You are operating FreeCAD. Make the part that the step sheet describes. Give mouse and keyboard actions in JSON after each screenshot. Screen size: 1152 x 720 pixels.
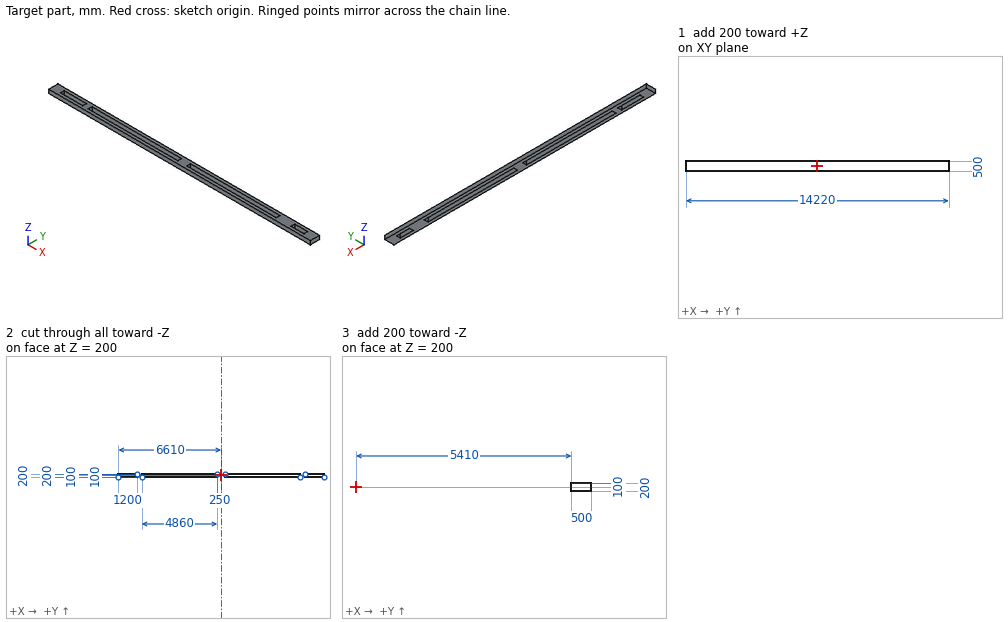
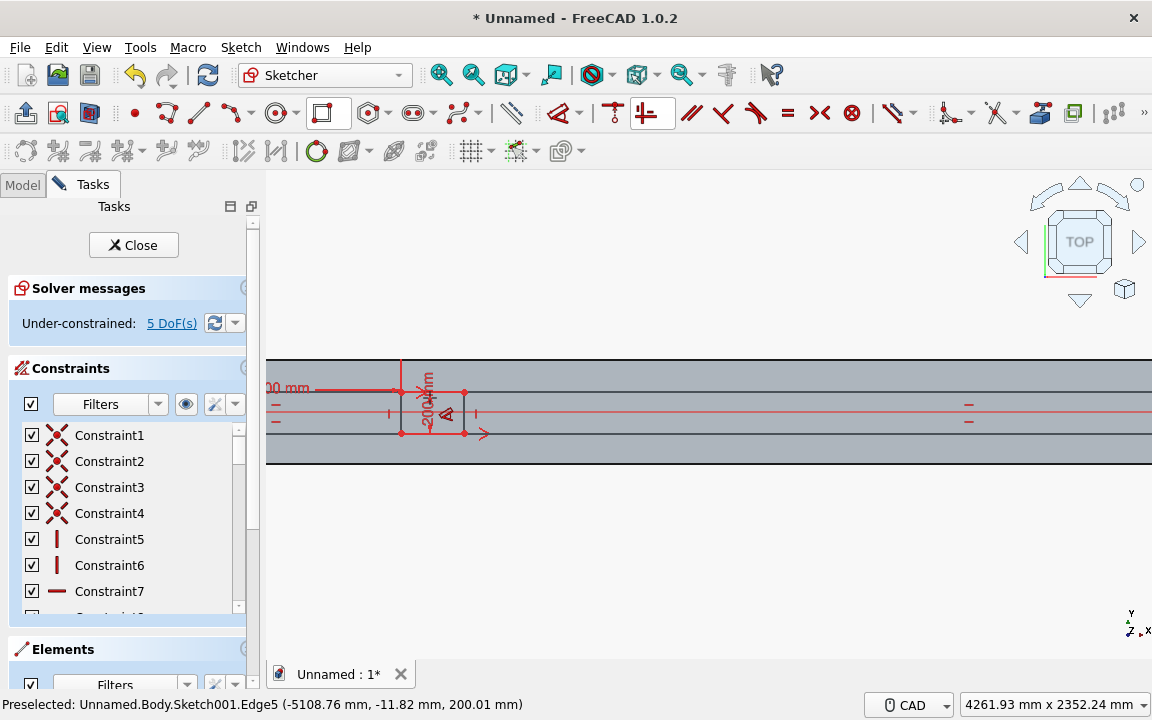
{"action": "left_click", "coordinate": [767, 434]}
{"action": "left_click", "coordinate": [726, 468]}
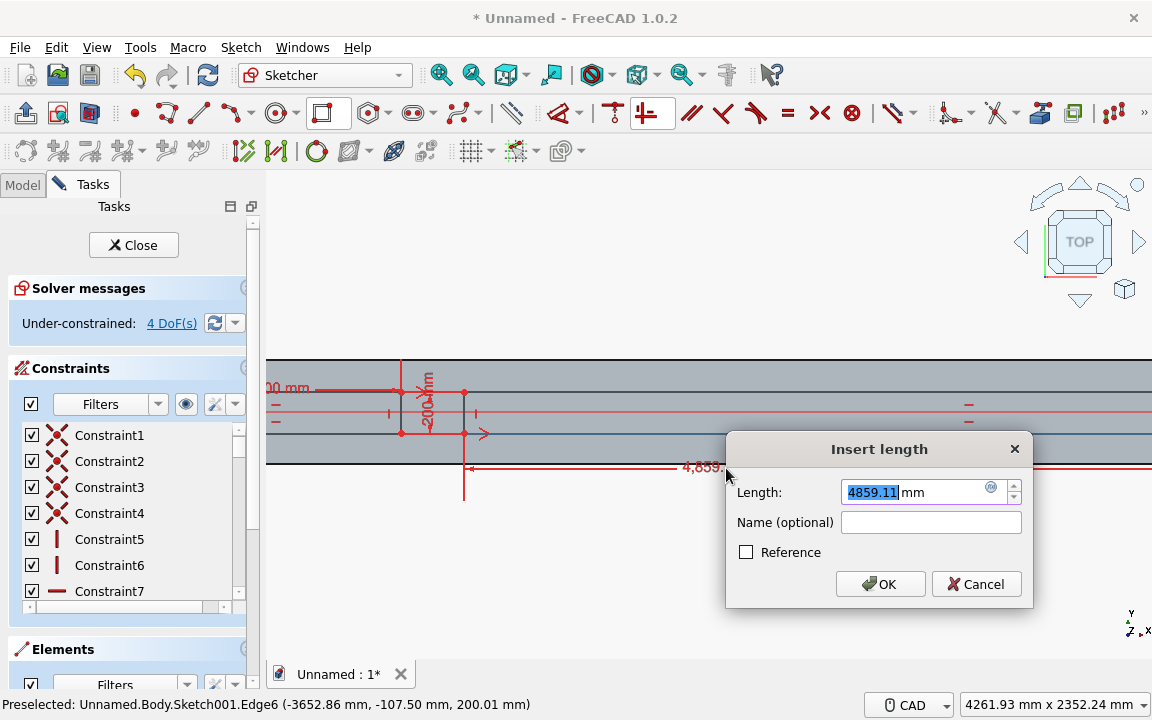
{"action": "type", "text": "4860"}
{"action": "key", "text": "Return"}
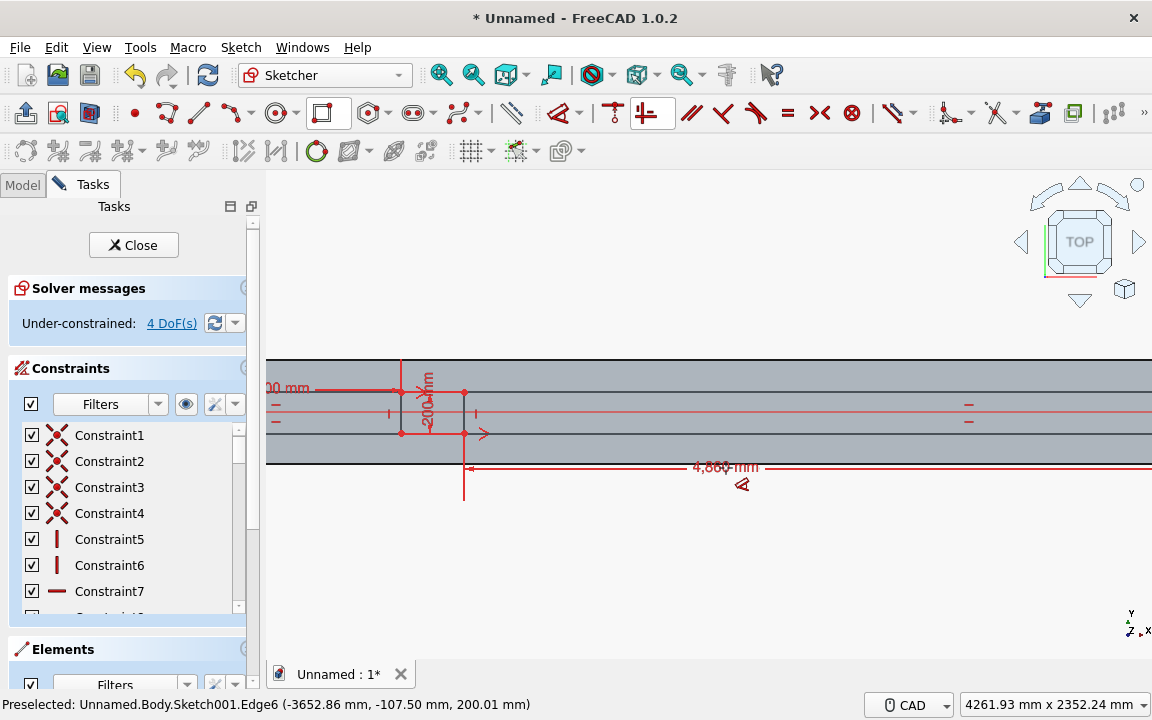
{"action": "scroll", "coordinate": [465, 415], "scroll_direction": "down", "scroll_amount": 9}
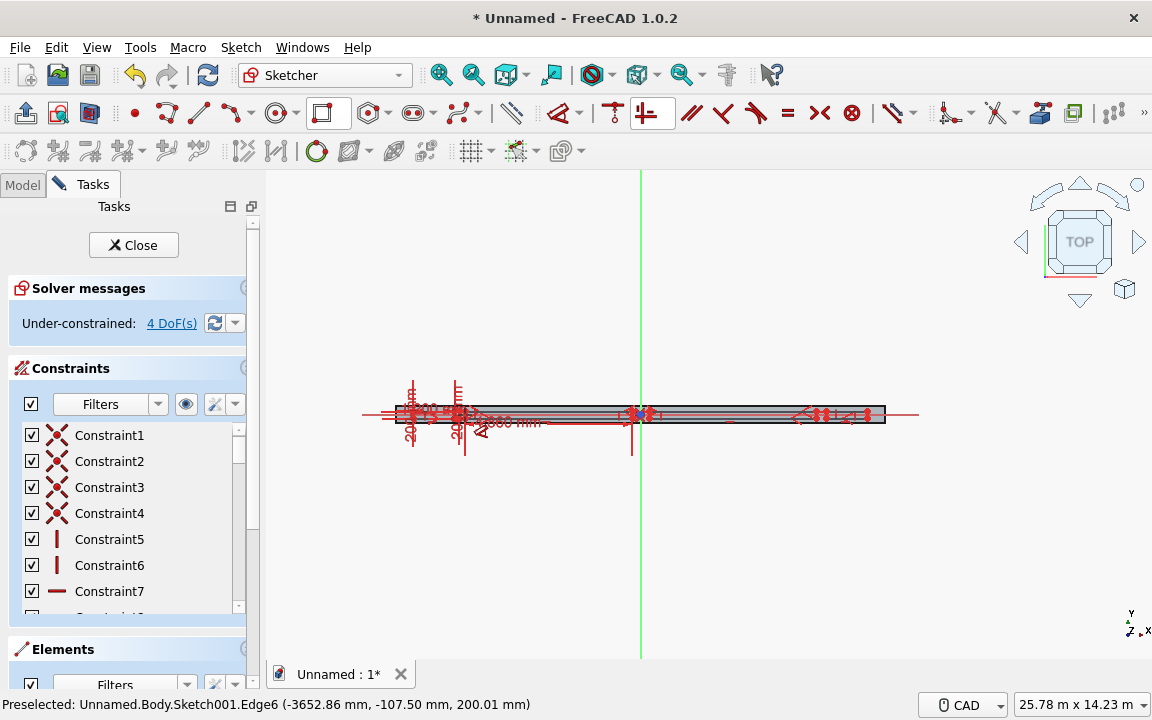
{"action": "scroll", "coordinate": [413, 412], "scroll_direction": "up", "scroll_amount": 13}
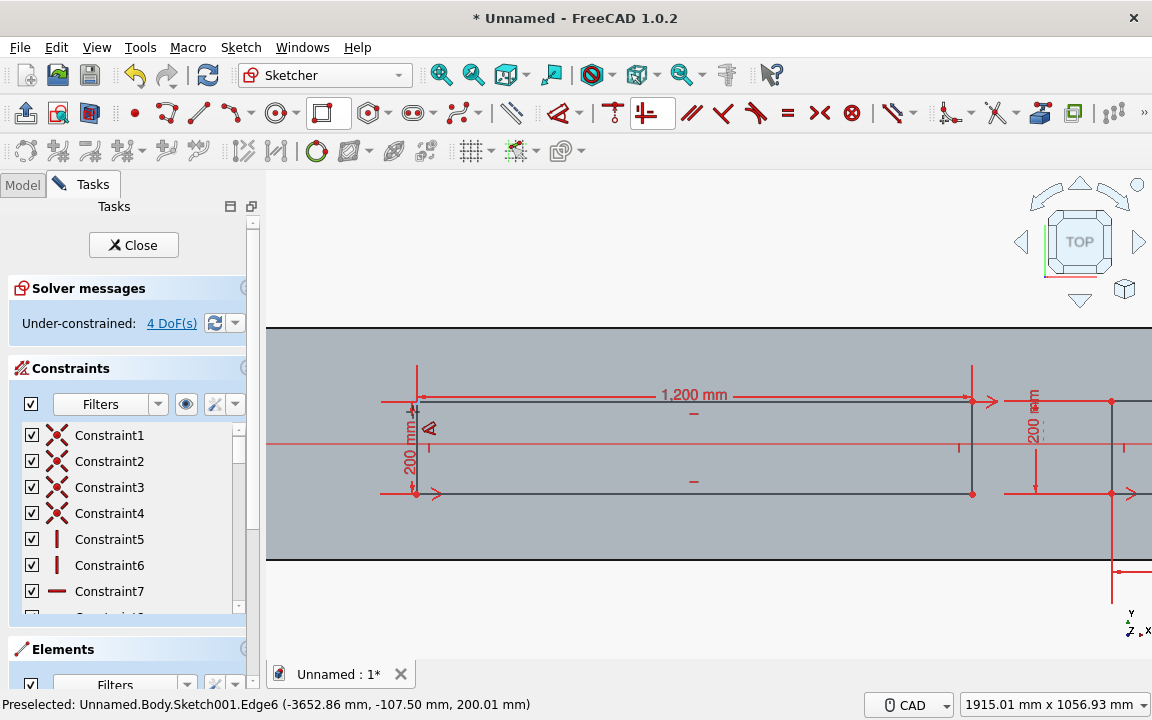
{"action": "left_click", "coordinate": [417, 402]}
{"action": "left_click", "coordinate": [383, 423]}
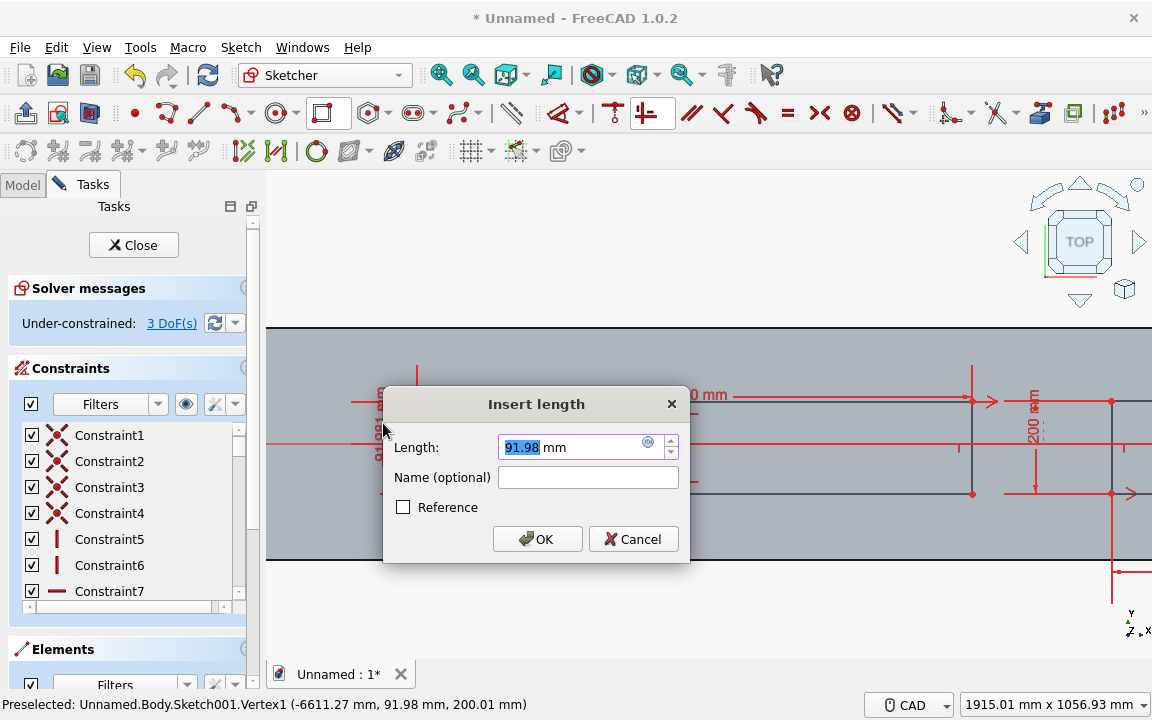
{"action": "type", "text": "100"}
{"action": "key", "text": "Return"}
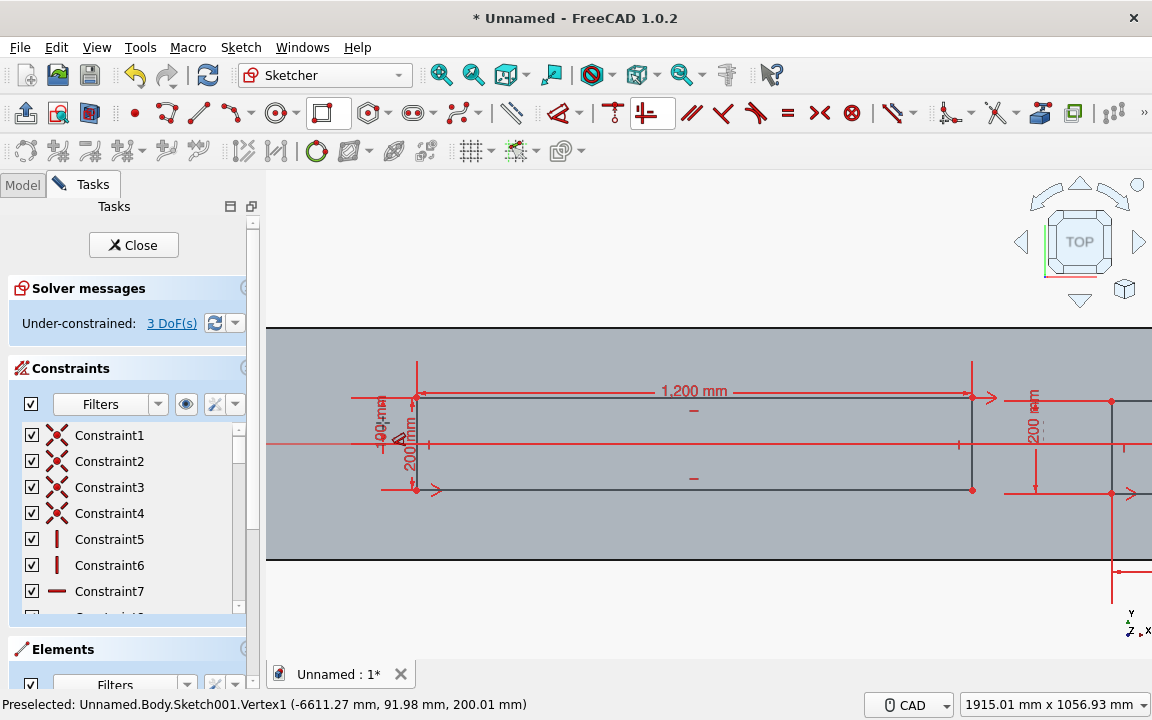
{"action": "scroll", "coordinate": [413, 412], "scroll_direction": "down", "scroll_amount": 13}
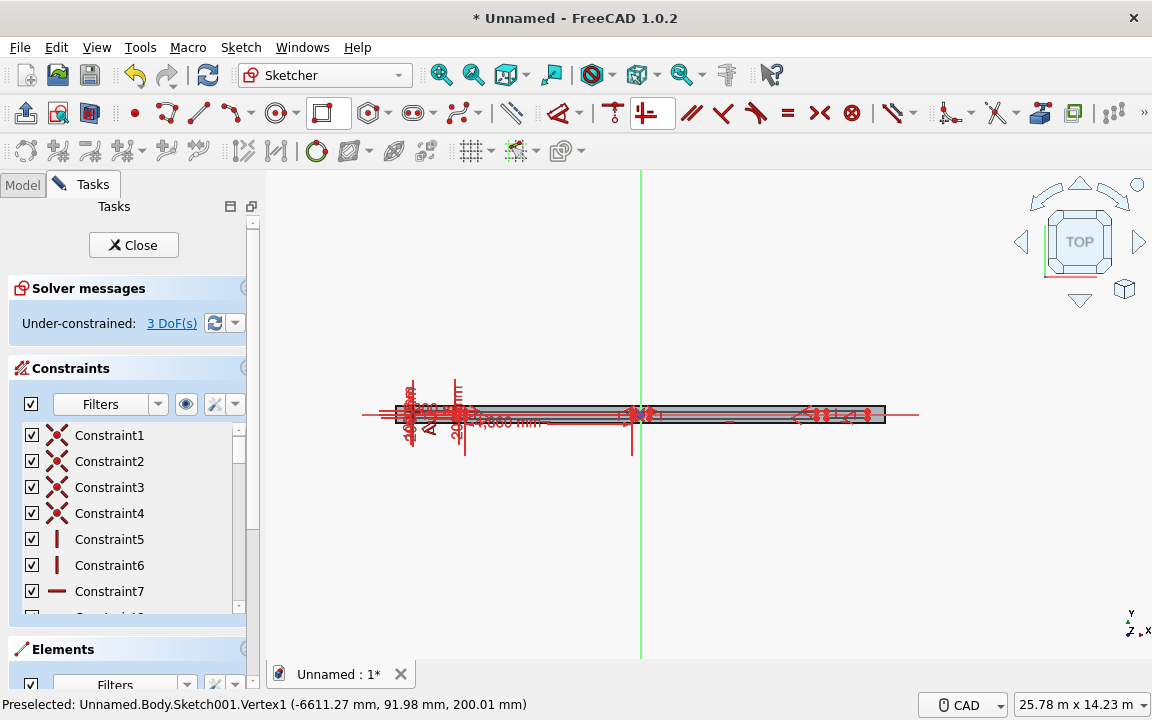
{"action": "scroll", "coordinate": [465, 412], "scroll_direction": "up", "scroll_amount": 13}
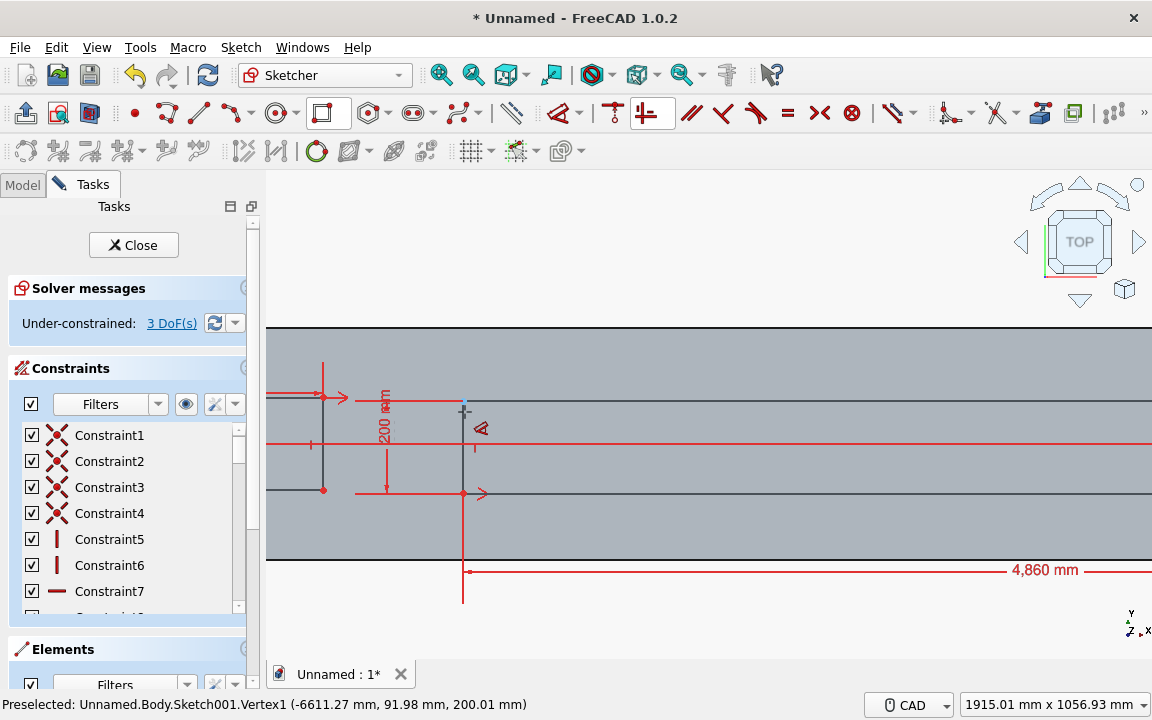
{"action": "left_click", "coordinate": [463, 401]}
{"action": "left_click", "coordinate": [309, 423]}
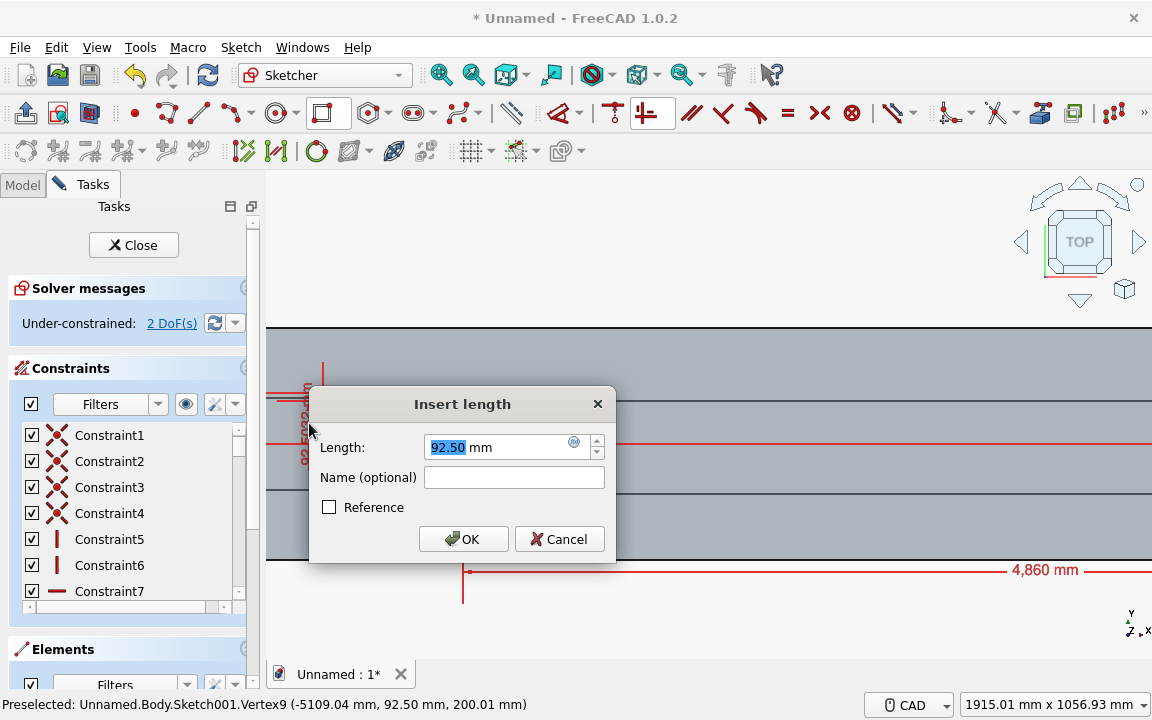
{"action": "type", "text": "100"}
{"action": "key", "text": "Return"}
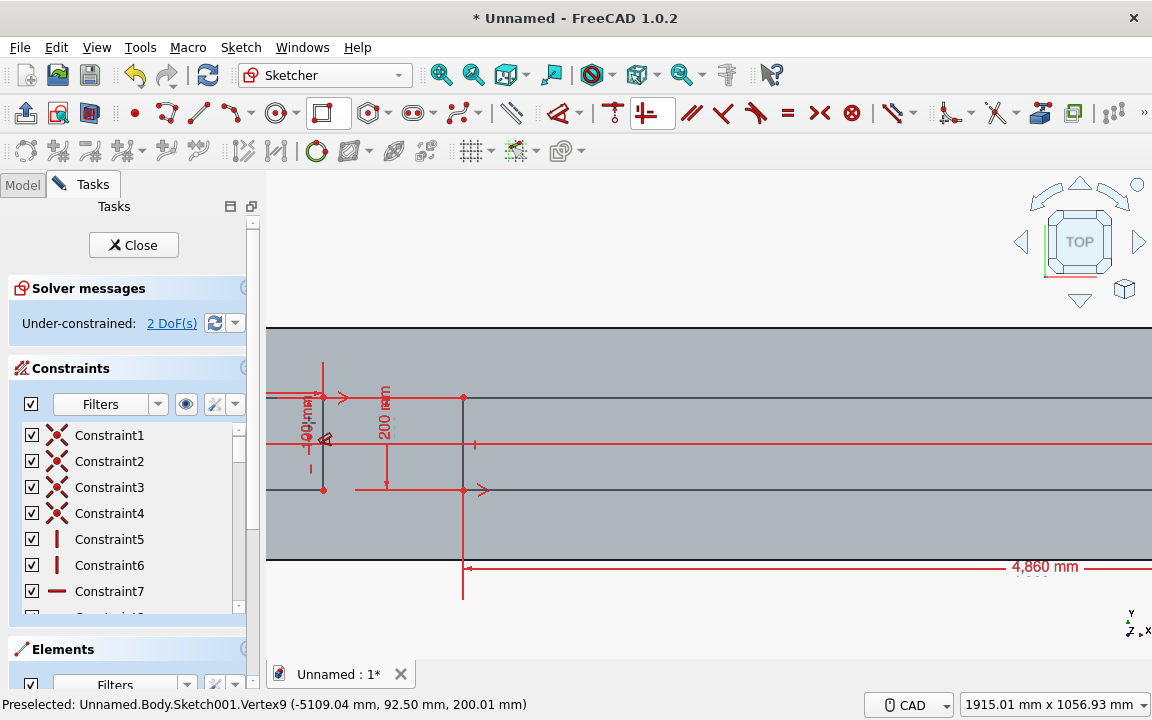
{"action": "scroll", "coordinate": [465, 412], "scroll_direction": "down", "scroll_amount": 13}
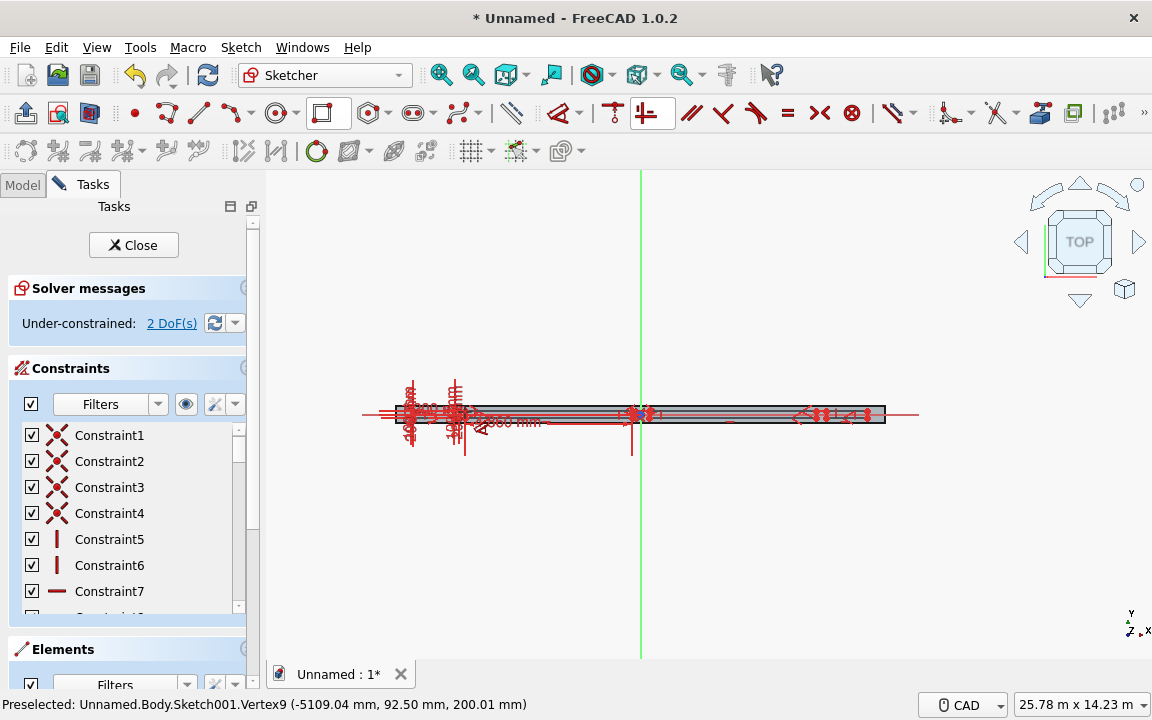
{"action": "scroll", "coordinate": [632, 418], "scroll_direction": "up", "scroll_amount": 8}